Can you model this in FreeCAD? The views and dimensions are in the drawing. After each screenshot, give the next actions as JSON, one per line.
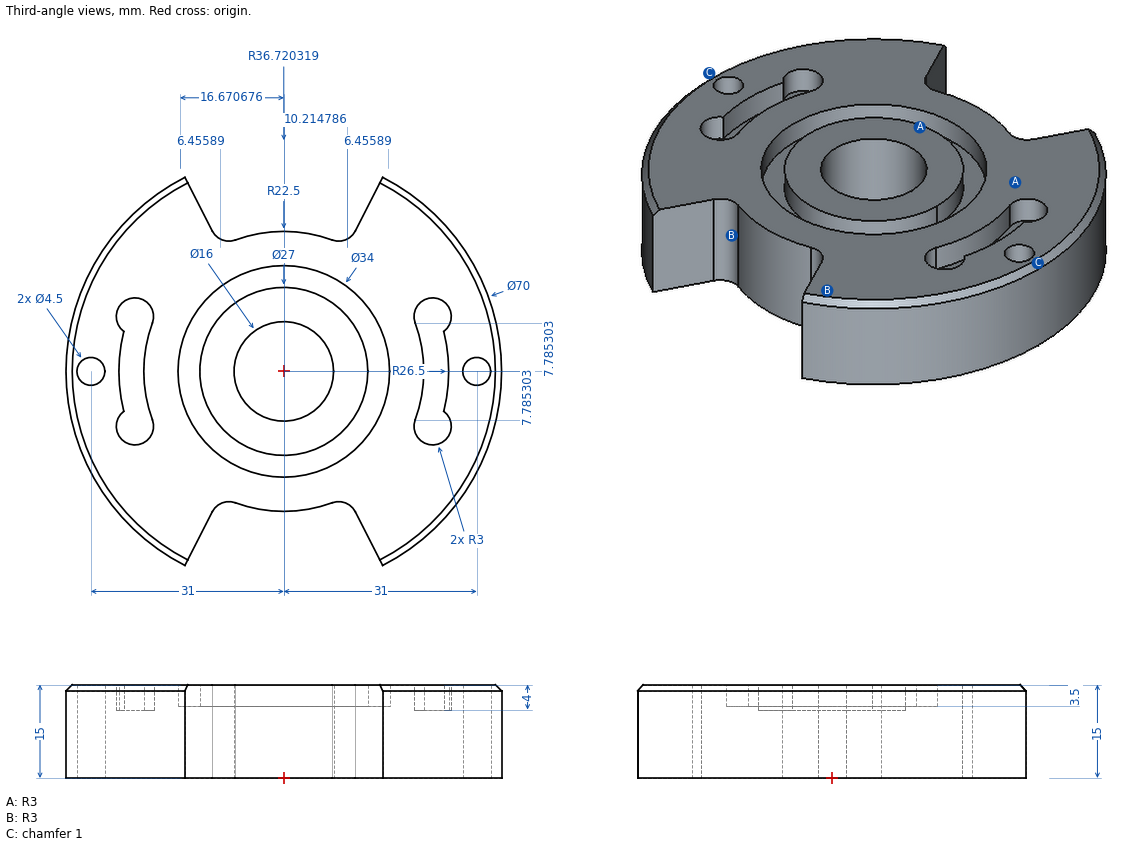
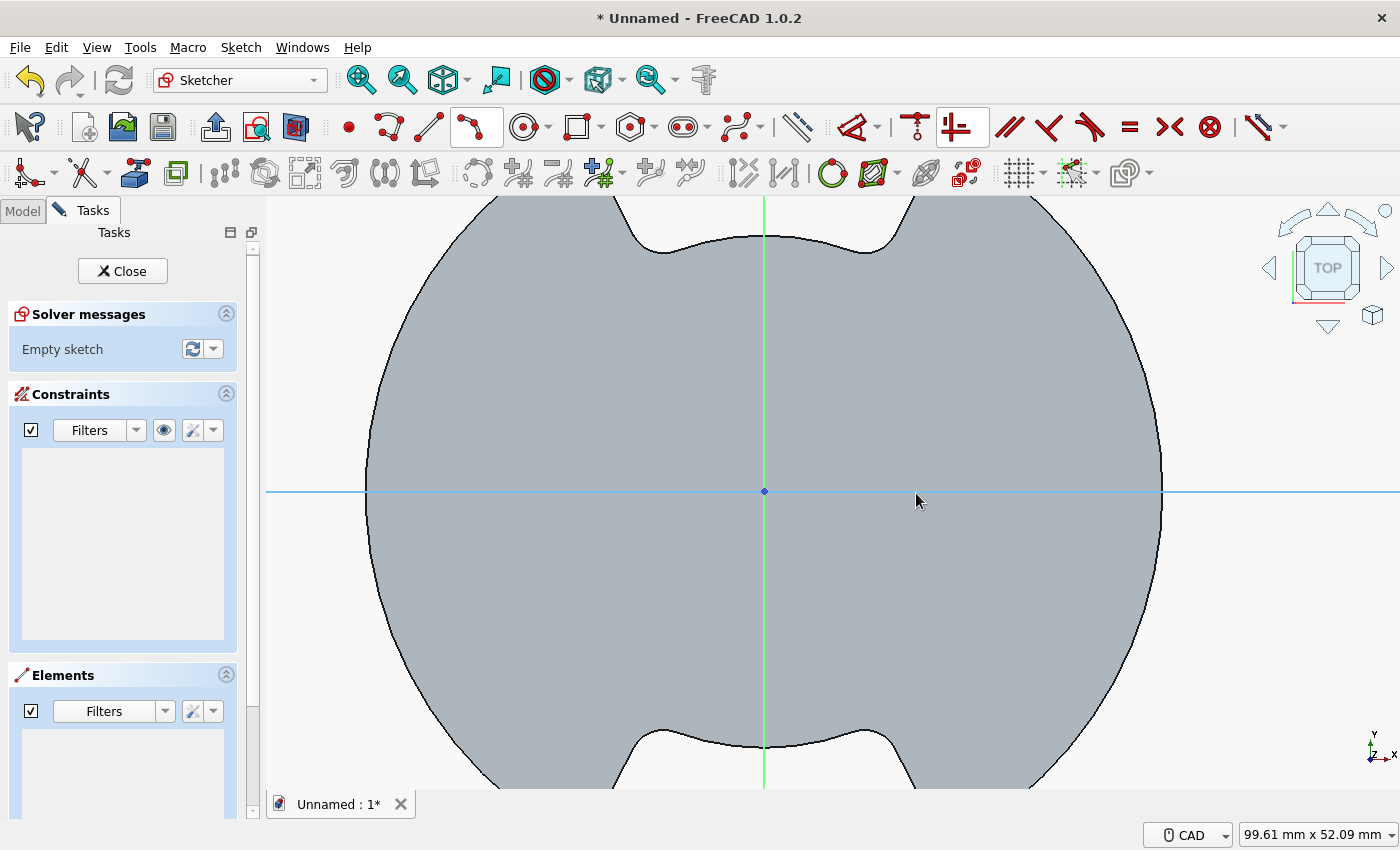
{"action": "key", "text": "g c"}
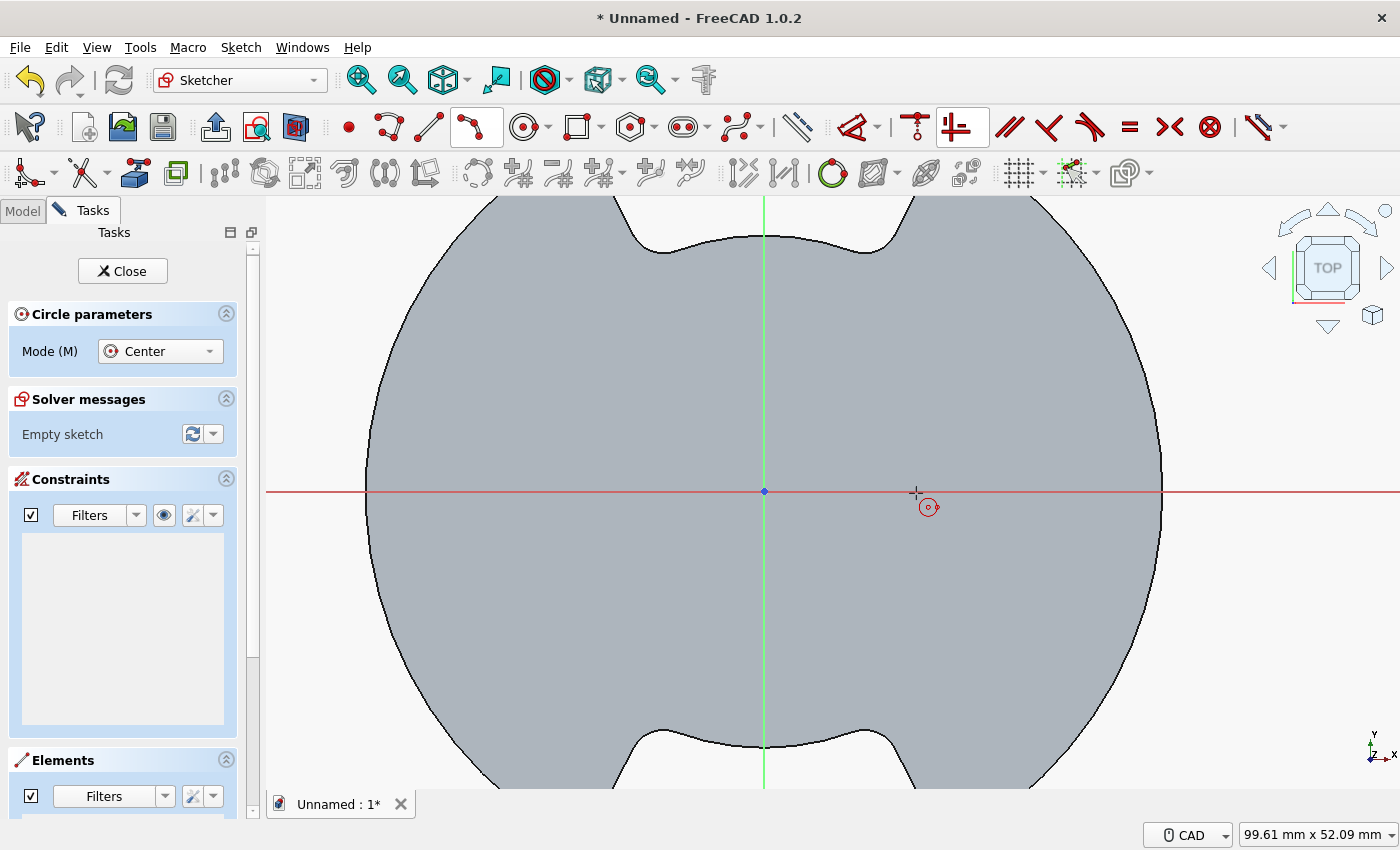
{"action": "left_click", "coordinate": [764, 492]}
{"action": "mouse_move", "coordinate": [901, 355]}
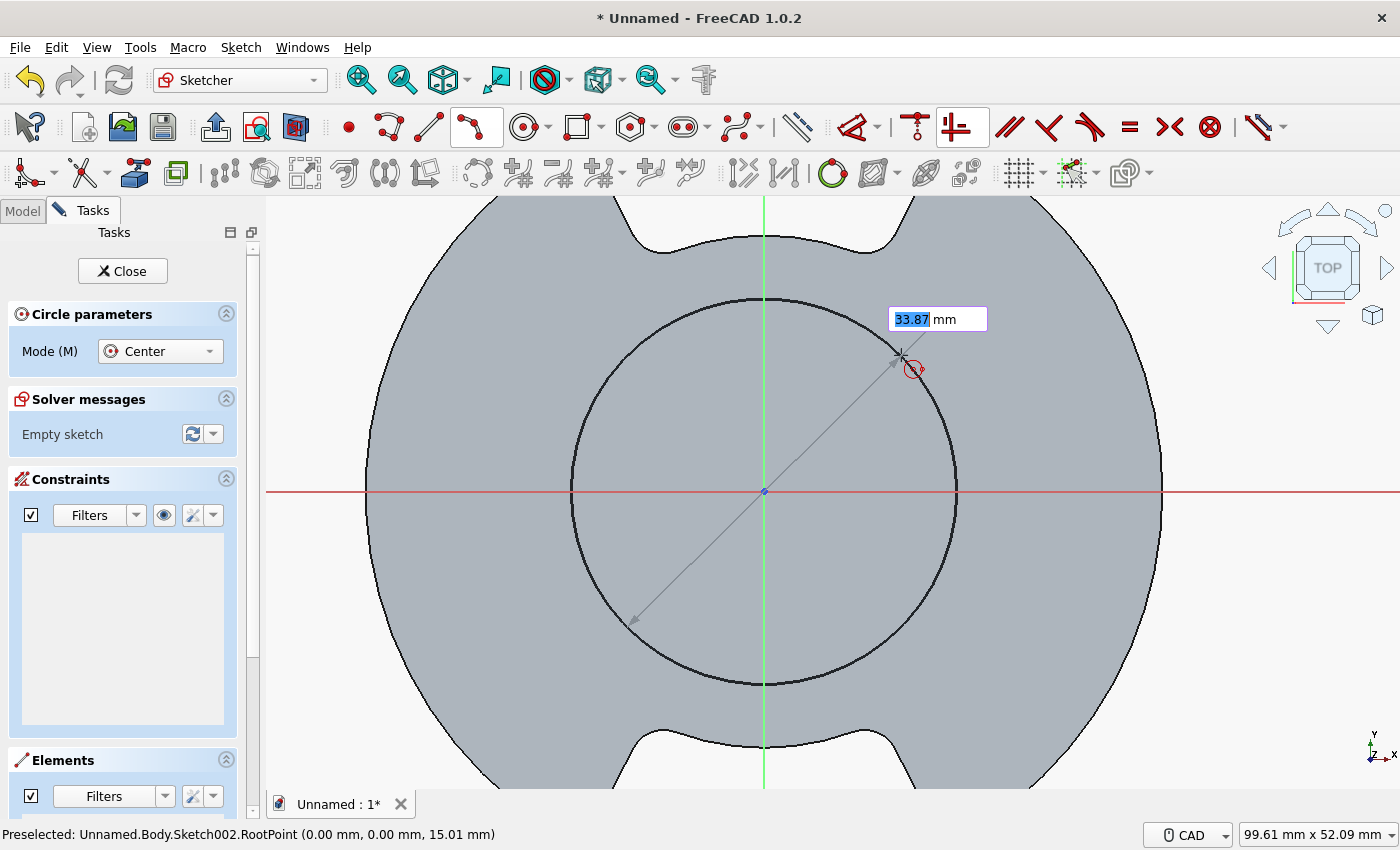
{"action": "type", "text": "34"}
{"action": "key", "text": "Return"}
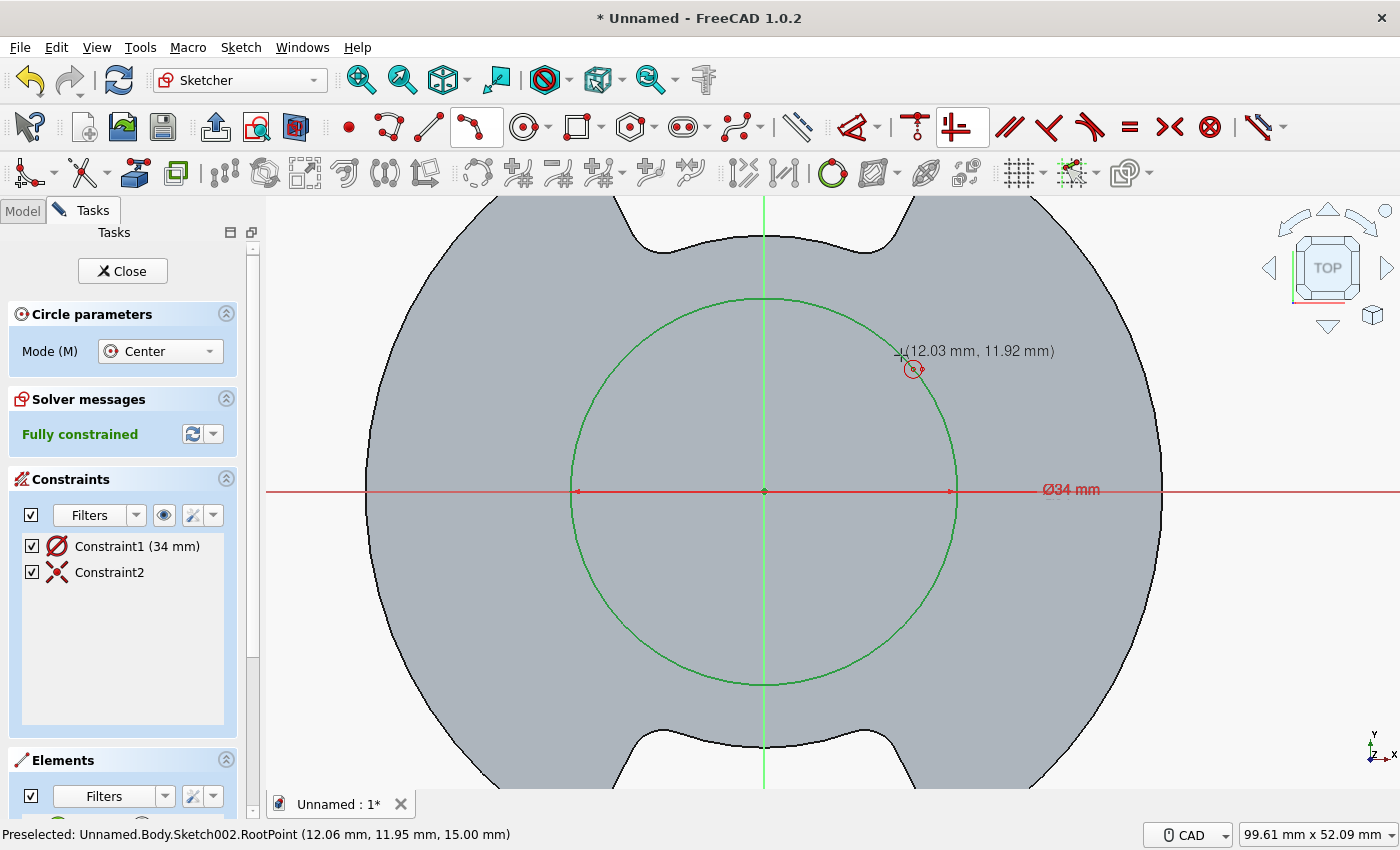
{"action": "left_click", "coordinate": [764, 492]}
{"action": "mouse_move", "coordinate": [873, 383]}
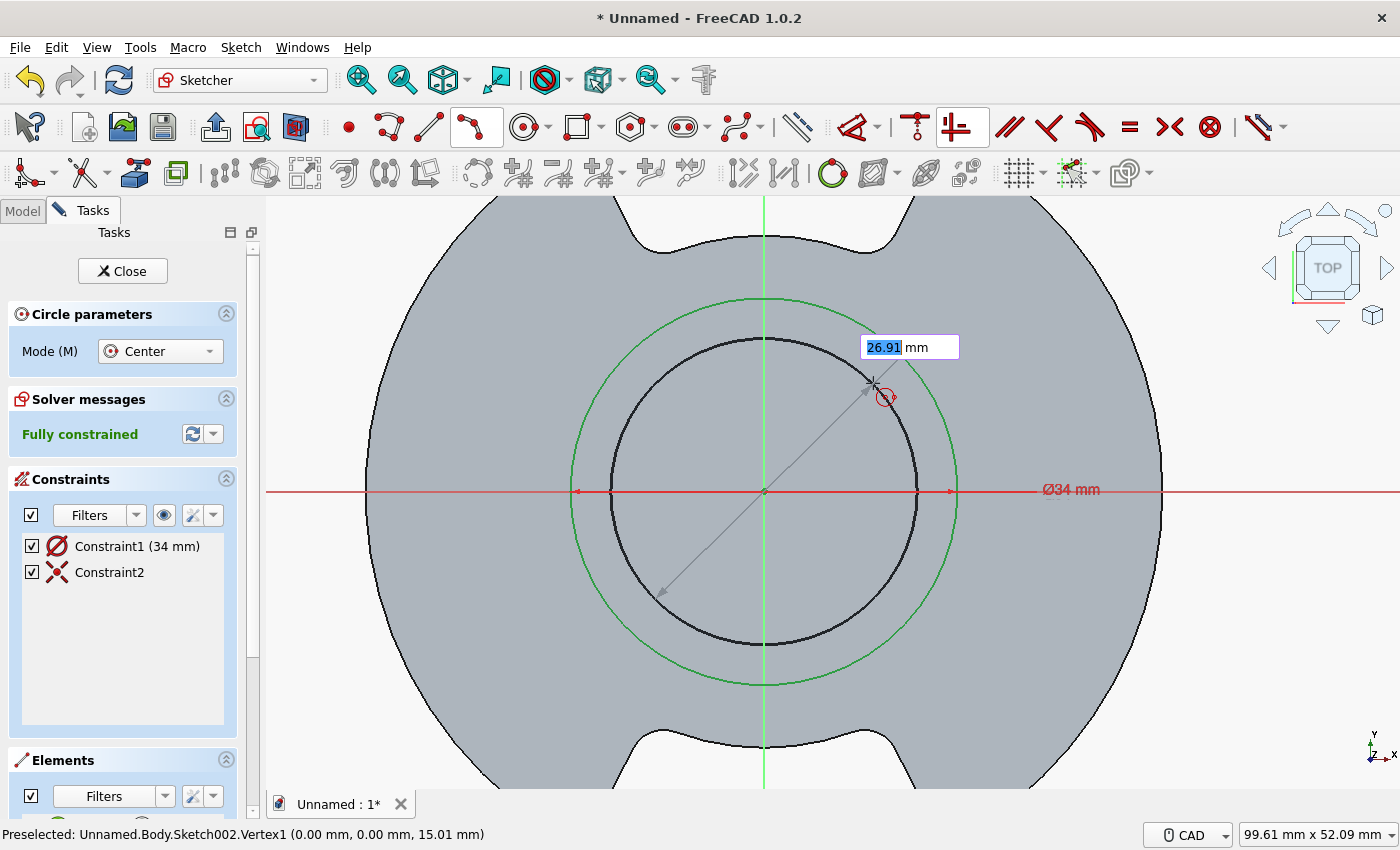
{"action": "type", "text": "27"}
{"action": "key", "text": "Return"}
{"action": "key", "text": "Escape"}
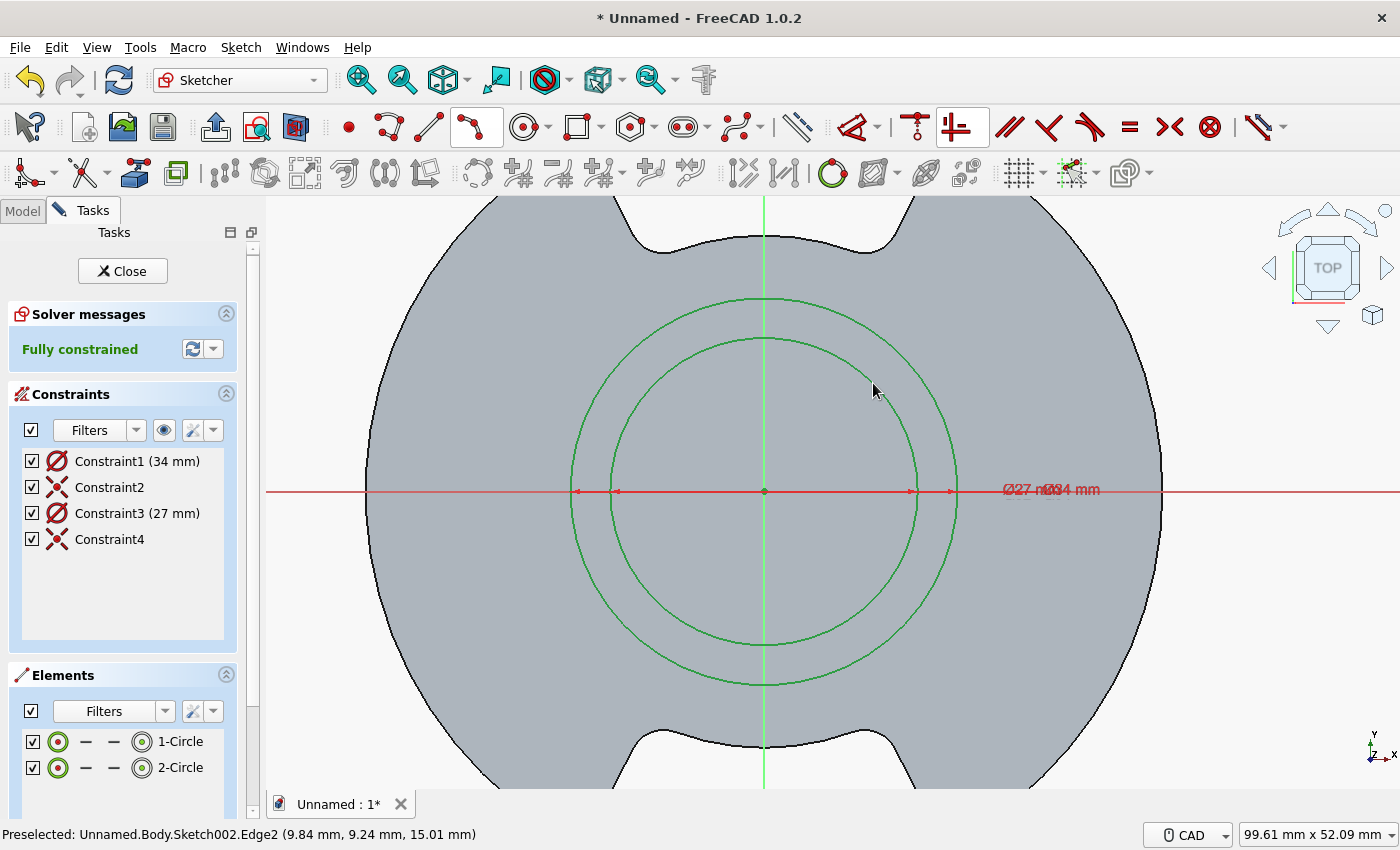
{"action": "left_click", "coordinate": [123, 271]}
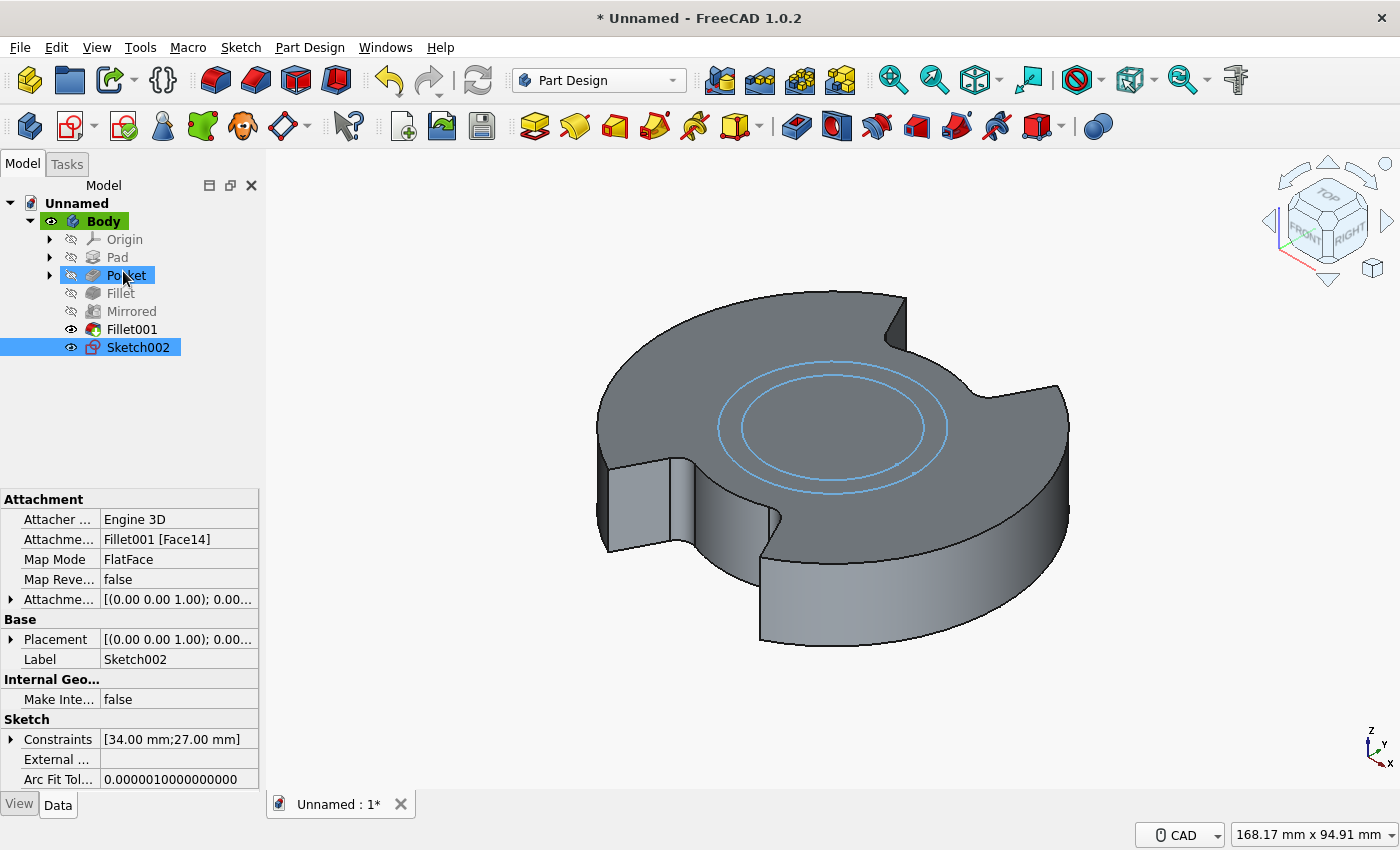
{"action": "left_click", "coordinate": [798, 126]}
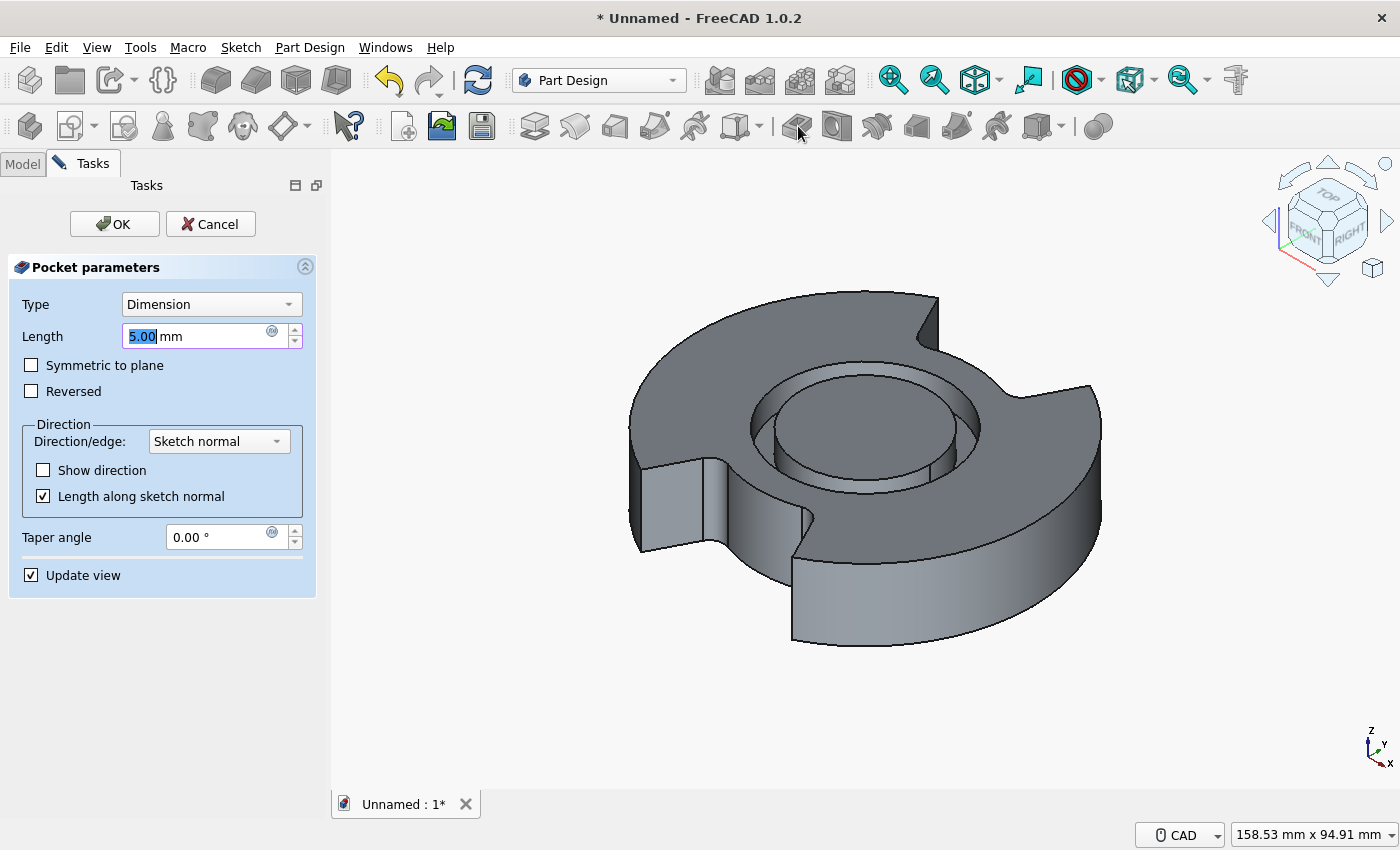
{"action": "type", "text": "3.5"}
{"action": "key", "text": "Tab"}